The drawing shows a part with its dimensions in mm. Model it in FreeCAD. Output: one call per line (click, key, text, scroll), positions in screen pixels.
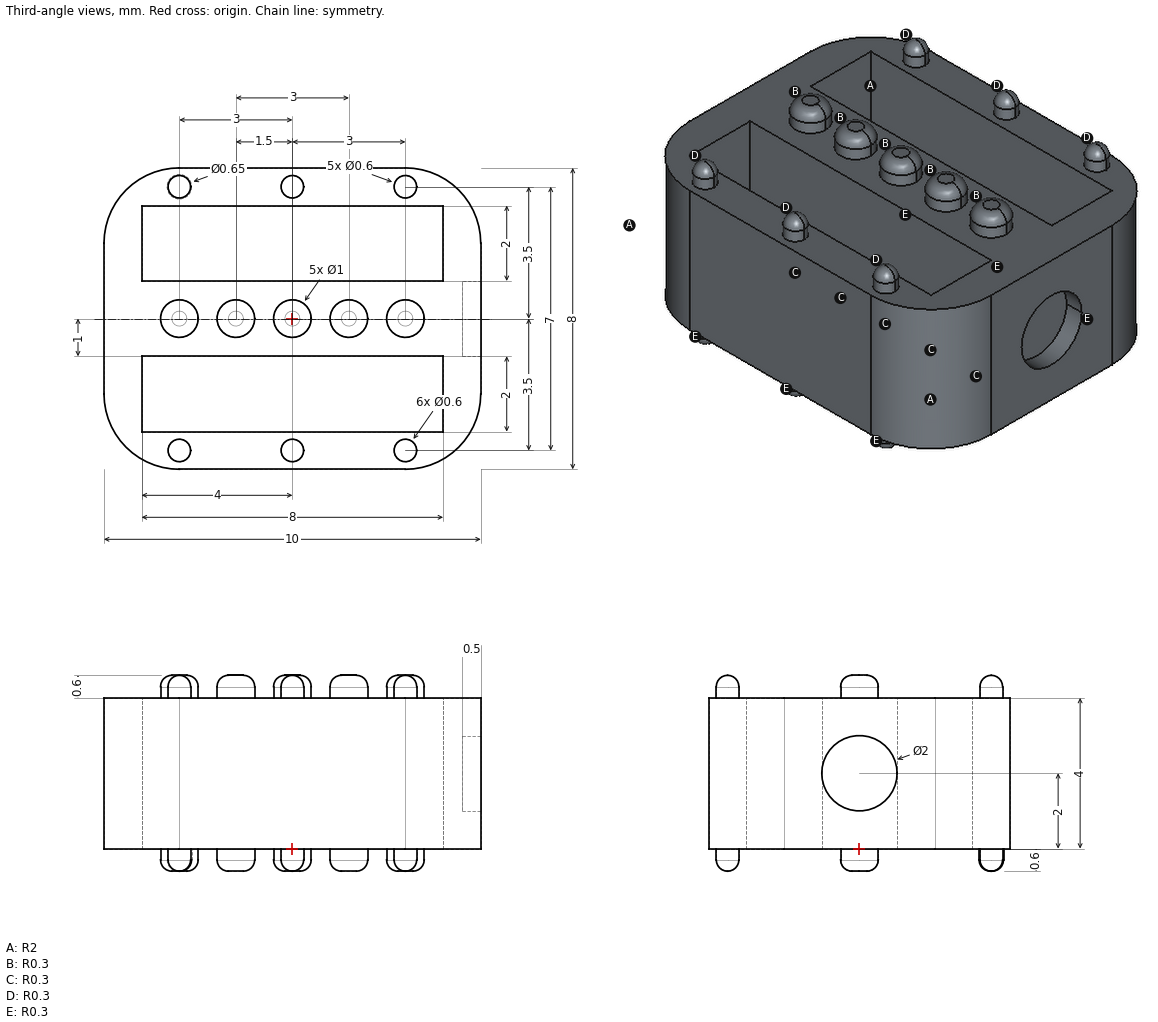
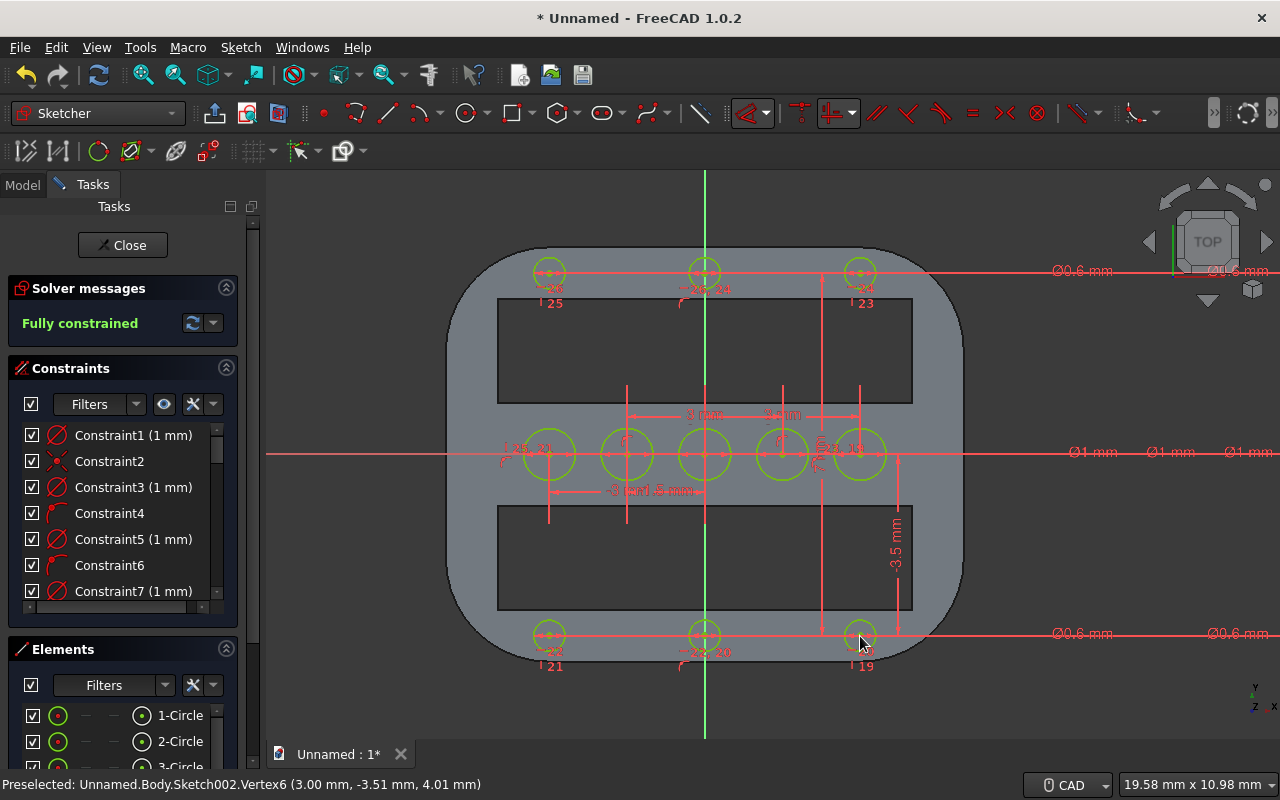
click(123, 245)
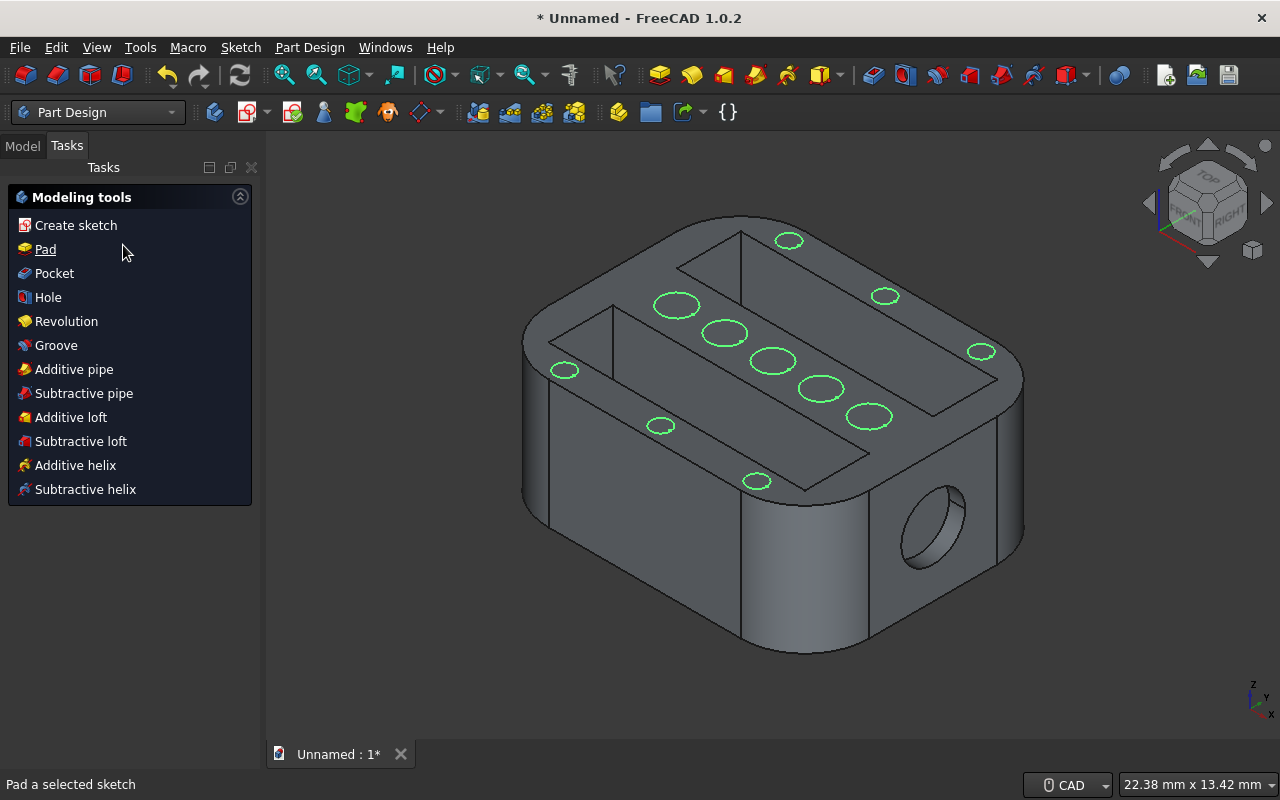
click(660, 76)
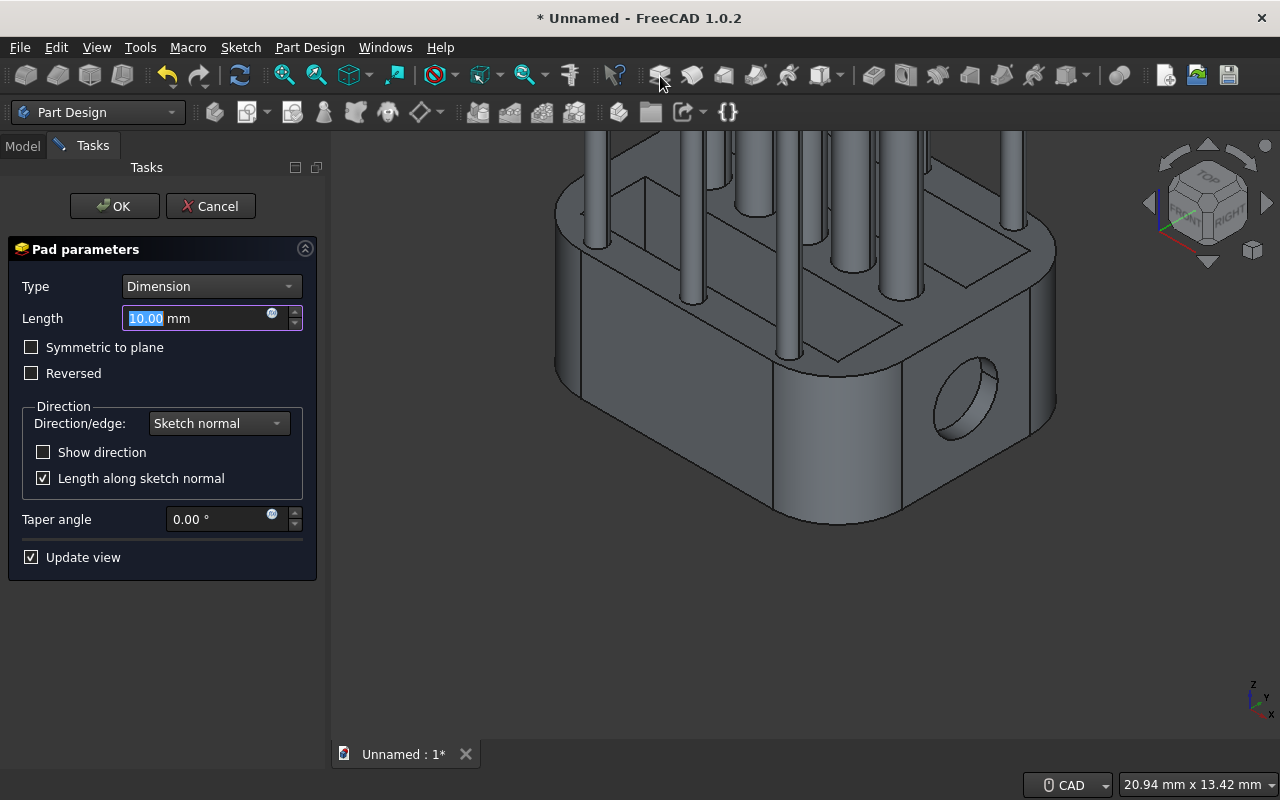
text(0.6)
key(Tab)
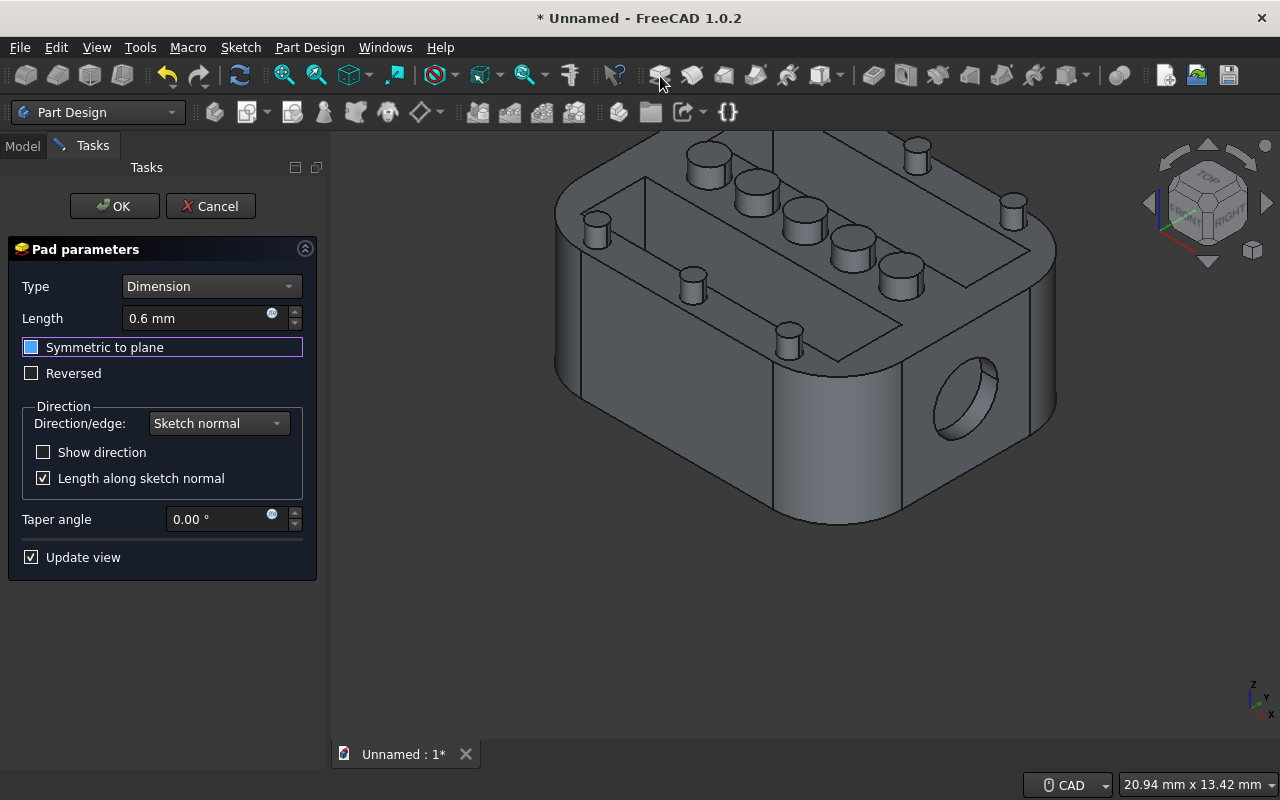
click(115, 206)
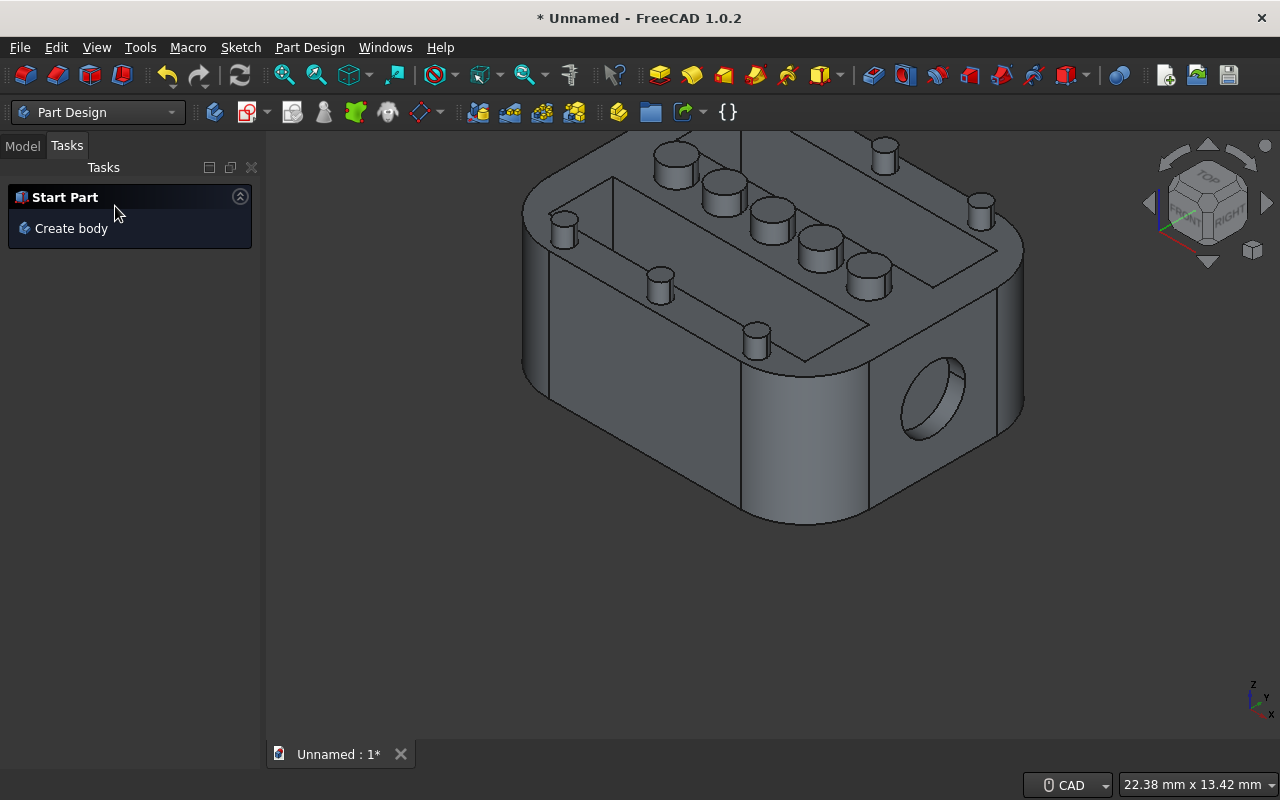
key(v)
key(f)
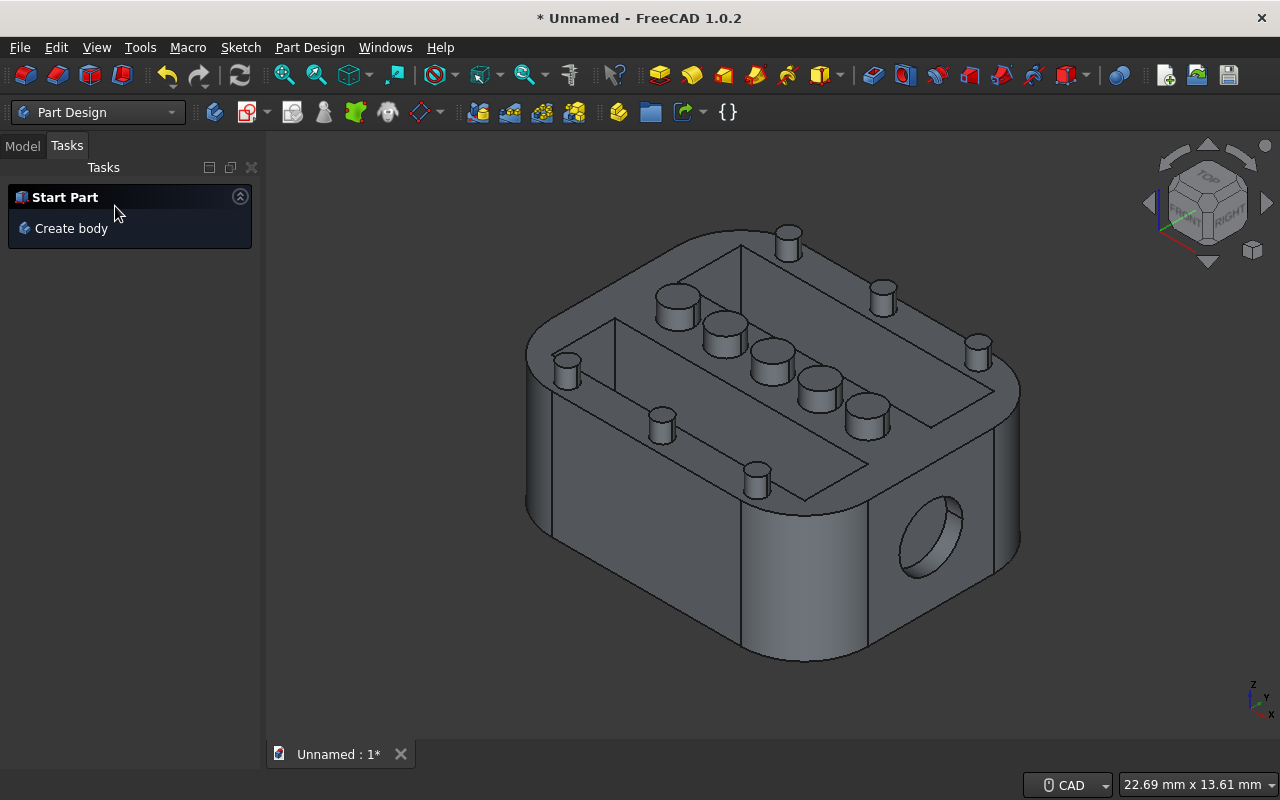
click(751, 348)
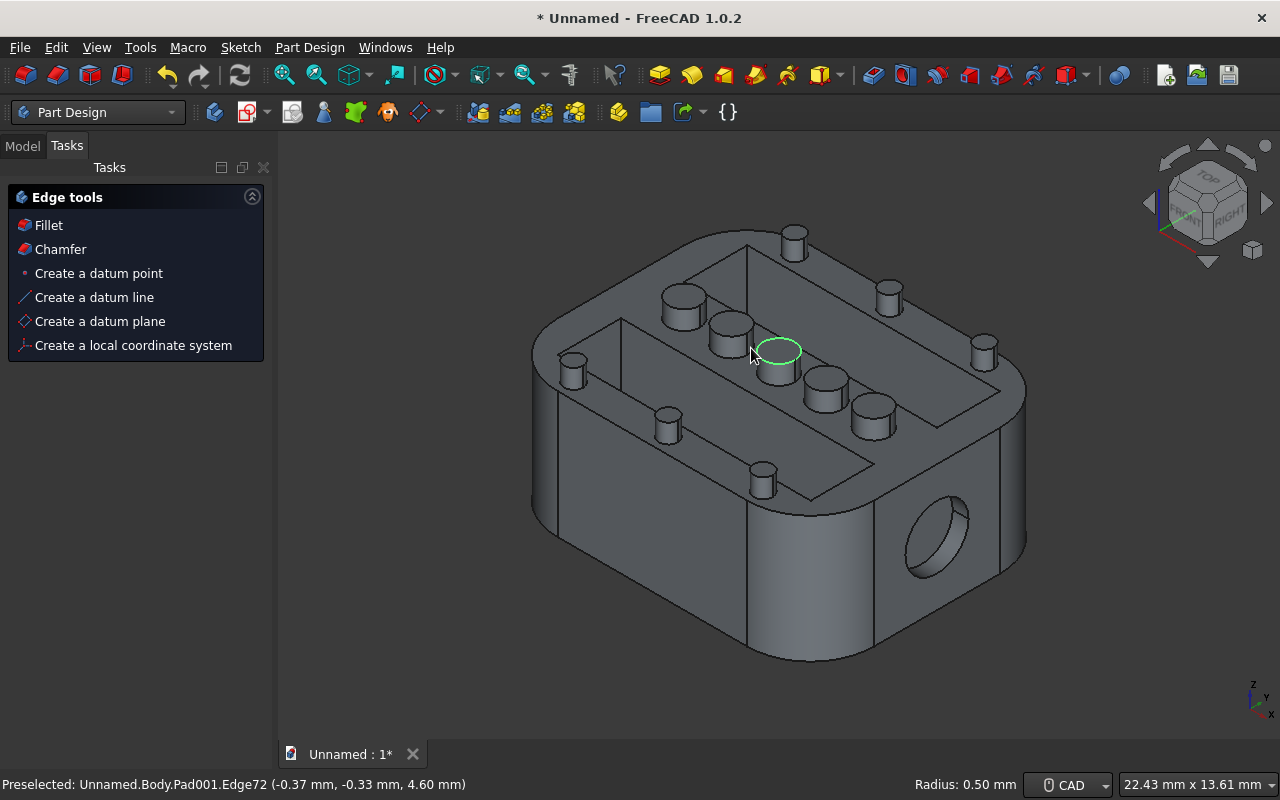
click(710, 321, ctrl)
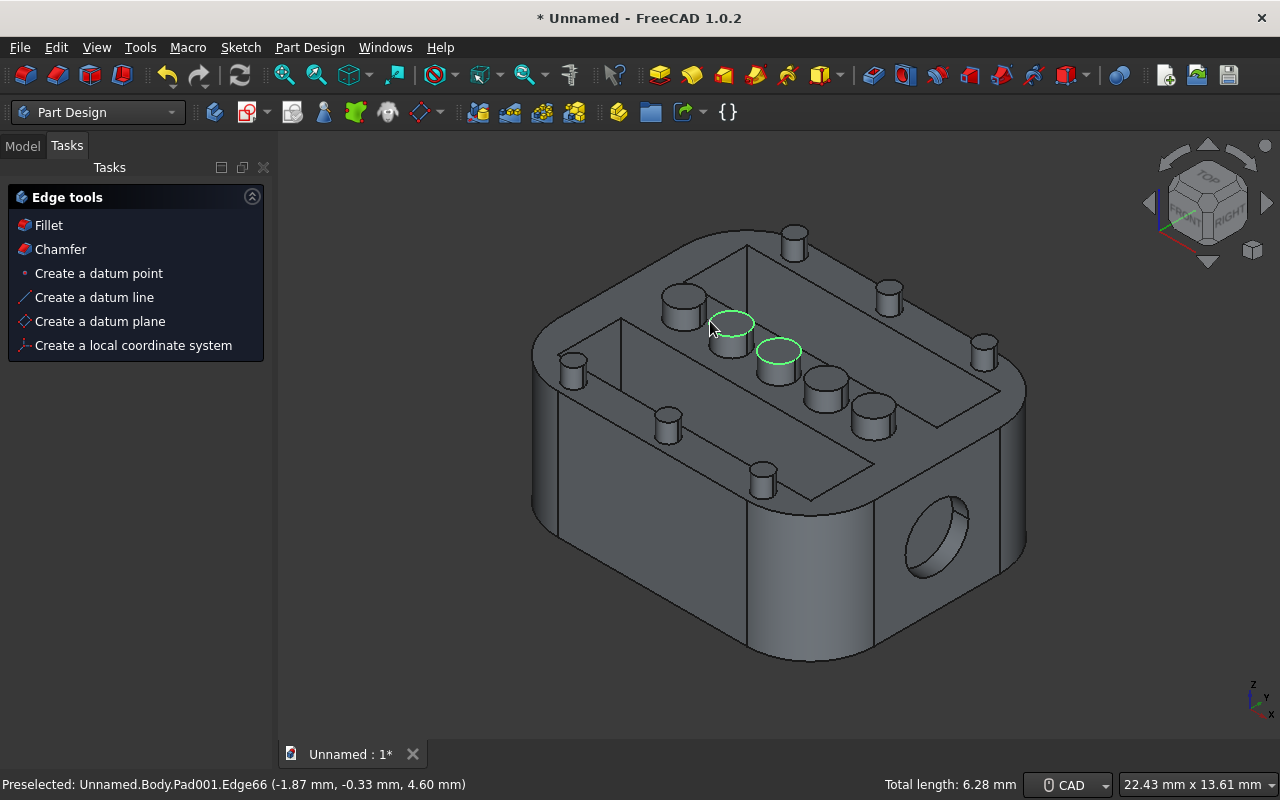
click(662, 293, ctrl)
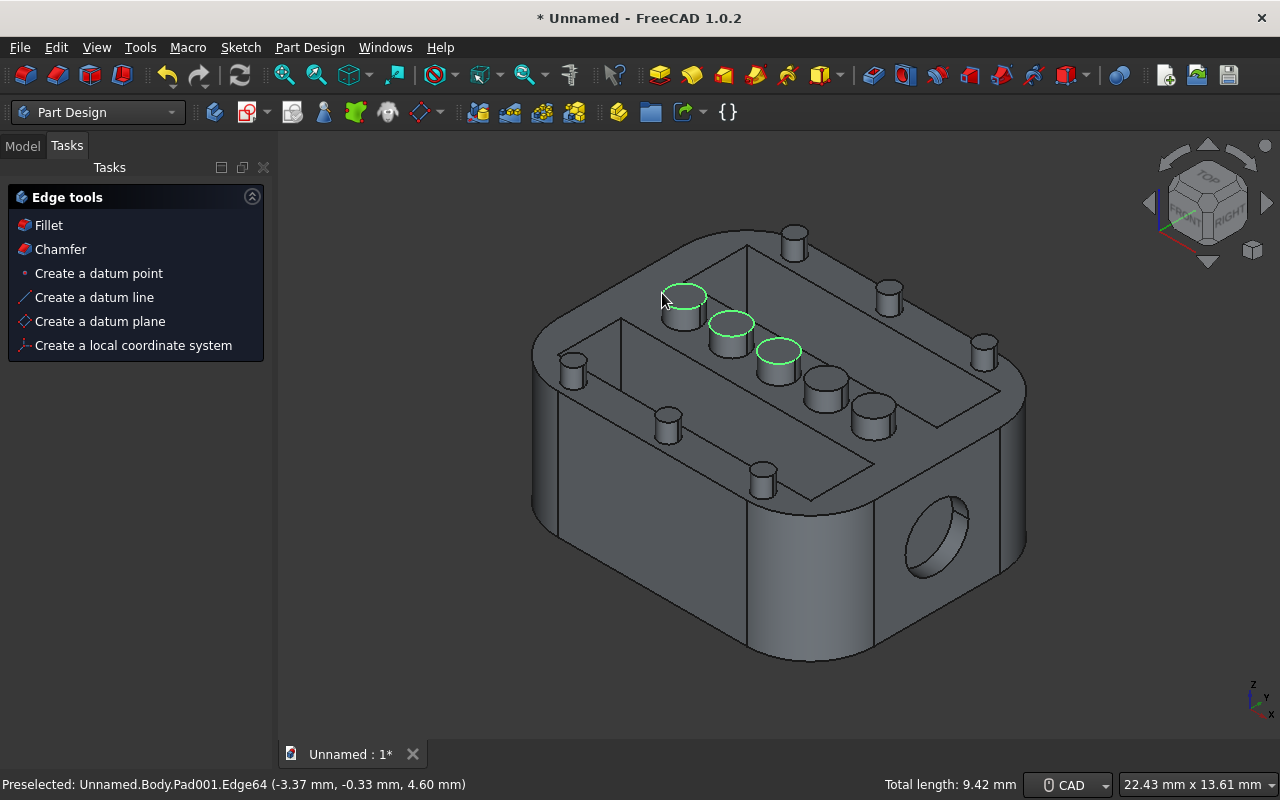
click(804, 375, ctrl)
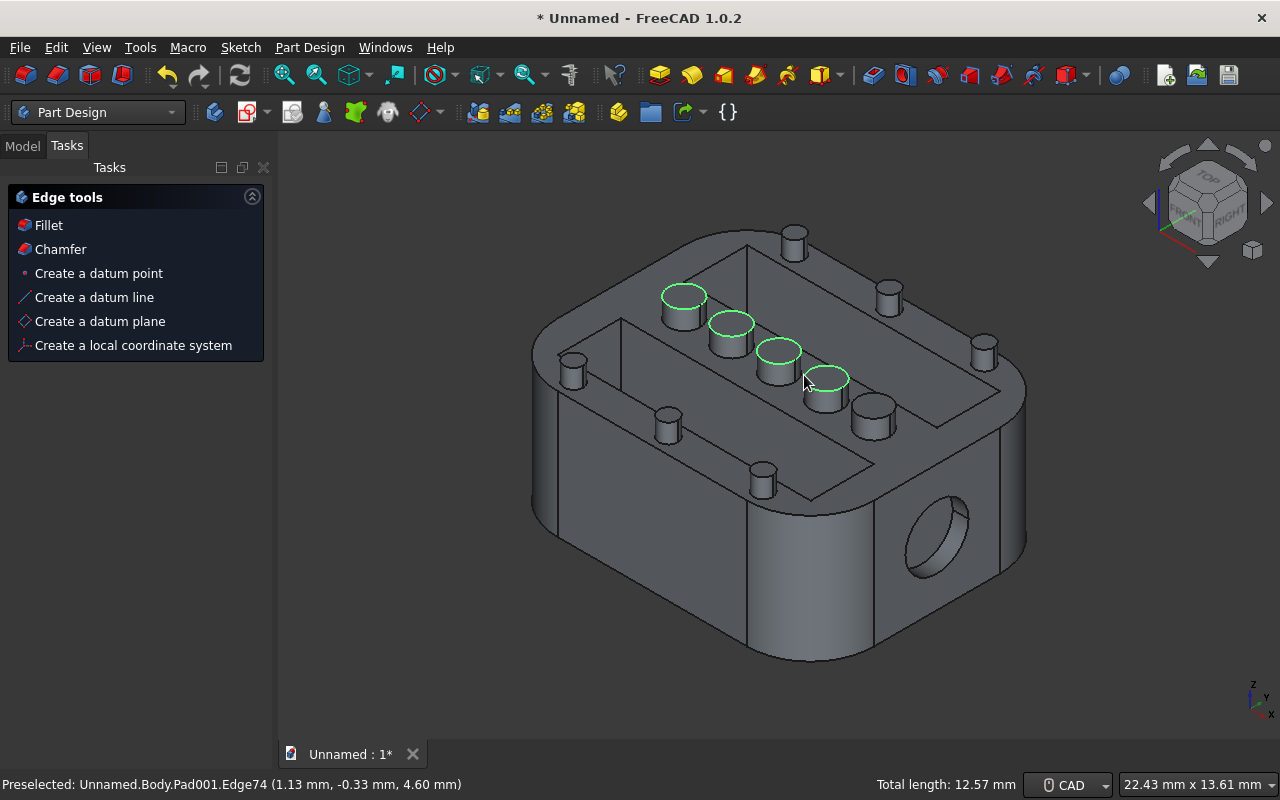
click(852, 403, ctrl)